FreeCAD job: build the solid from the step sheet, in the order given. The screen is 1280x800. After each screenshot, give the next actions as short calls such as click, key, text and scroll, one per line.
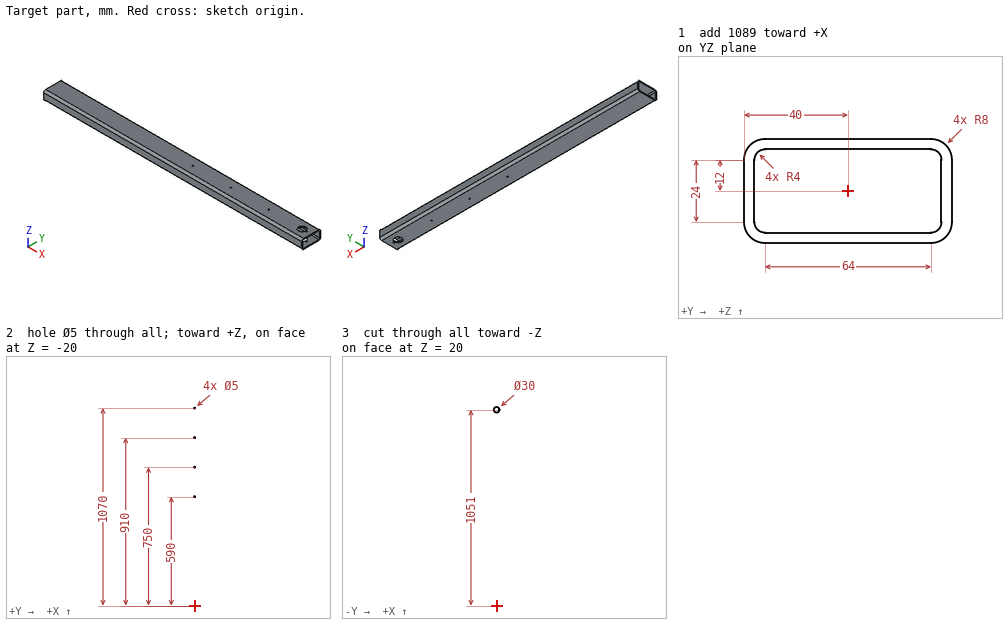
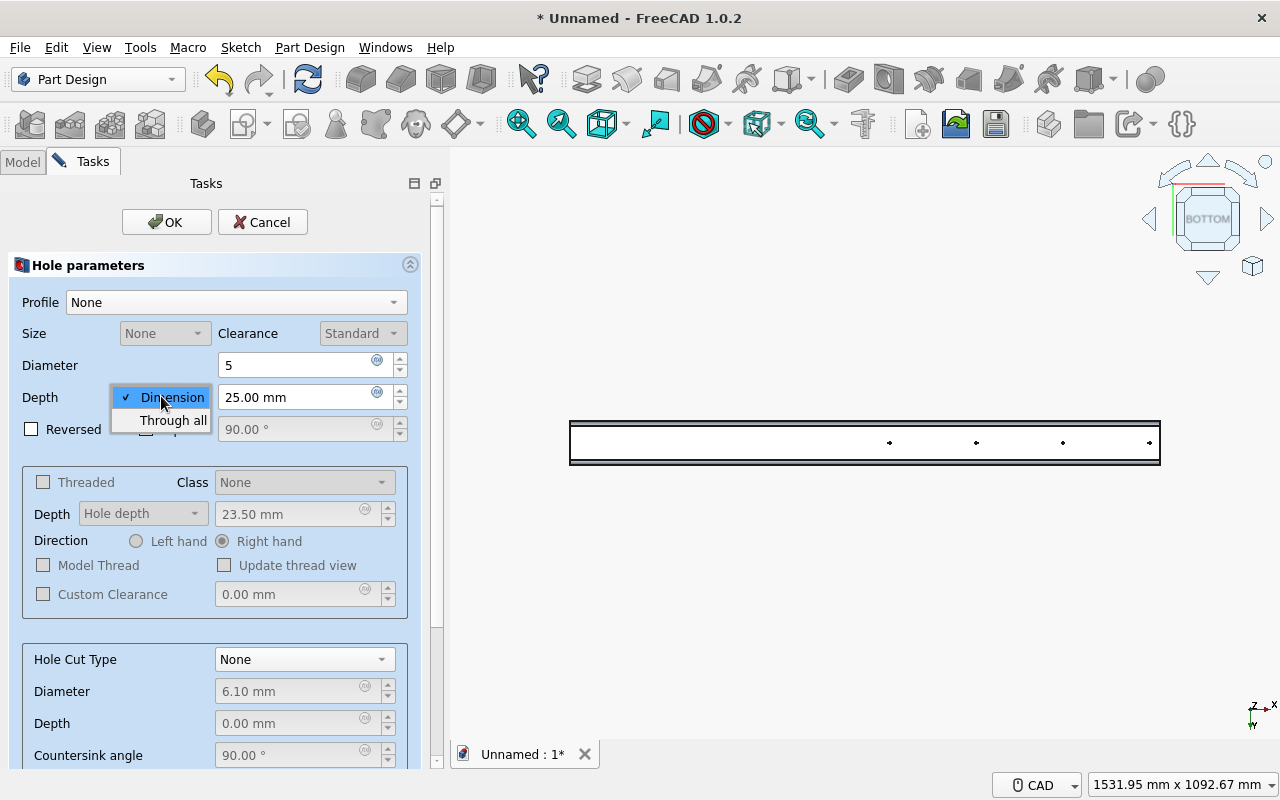
click(160, 420)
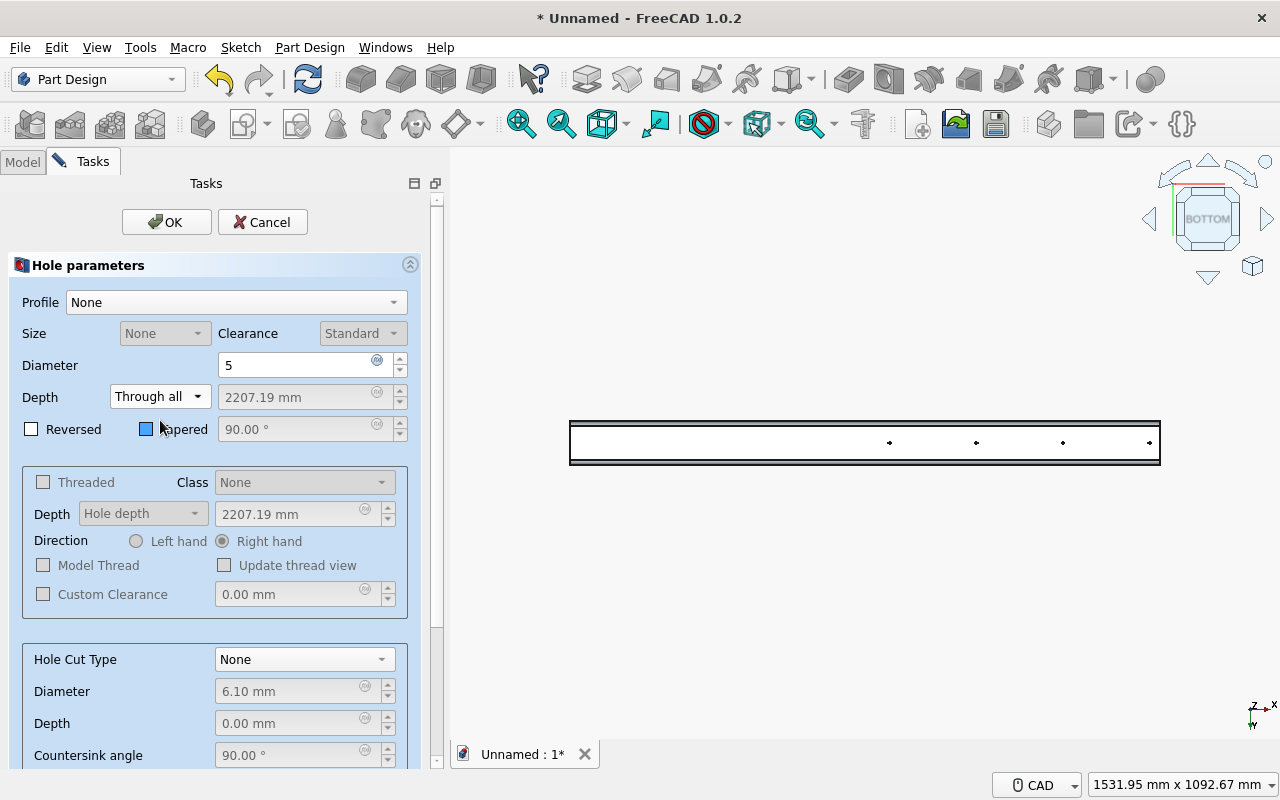
click(167, 222)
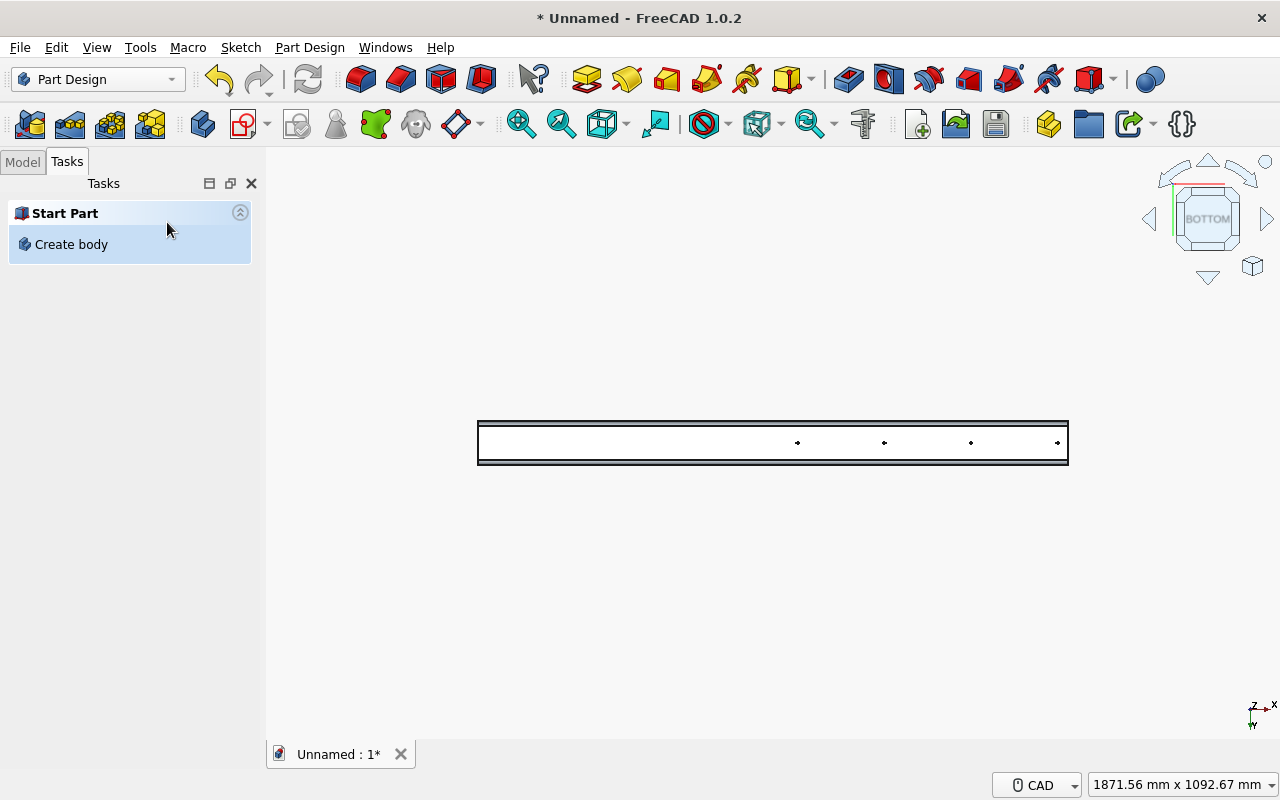
key(0)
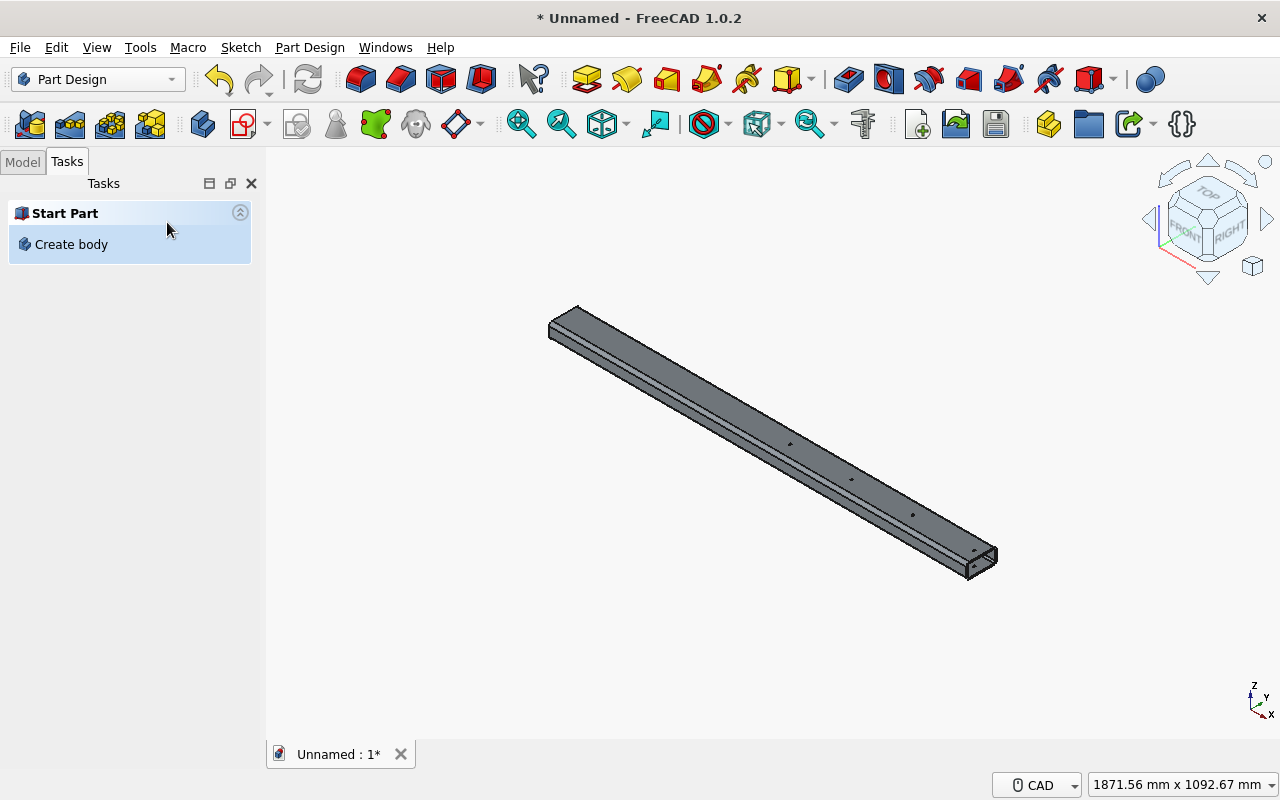
click(773, 433)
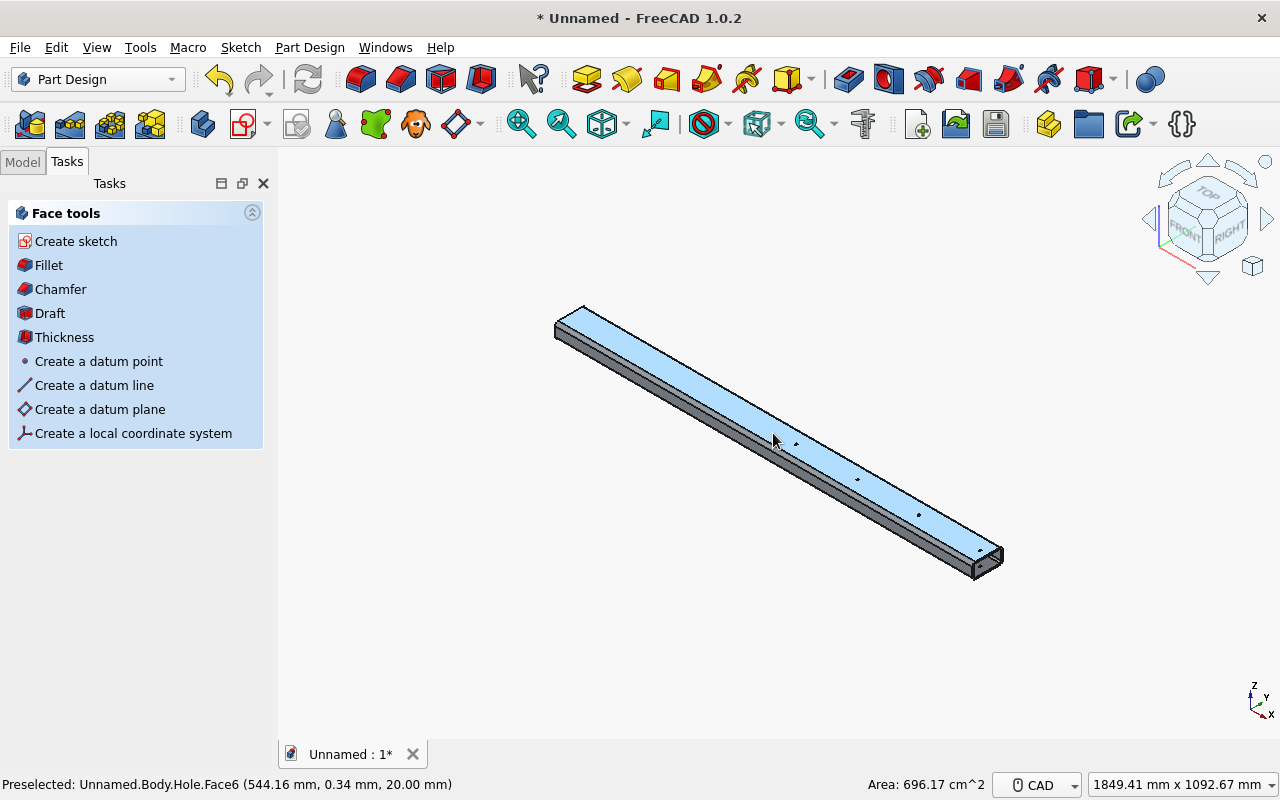
click(244, 124)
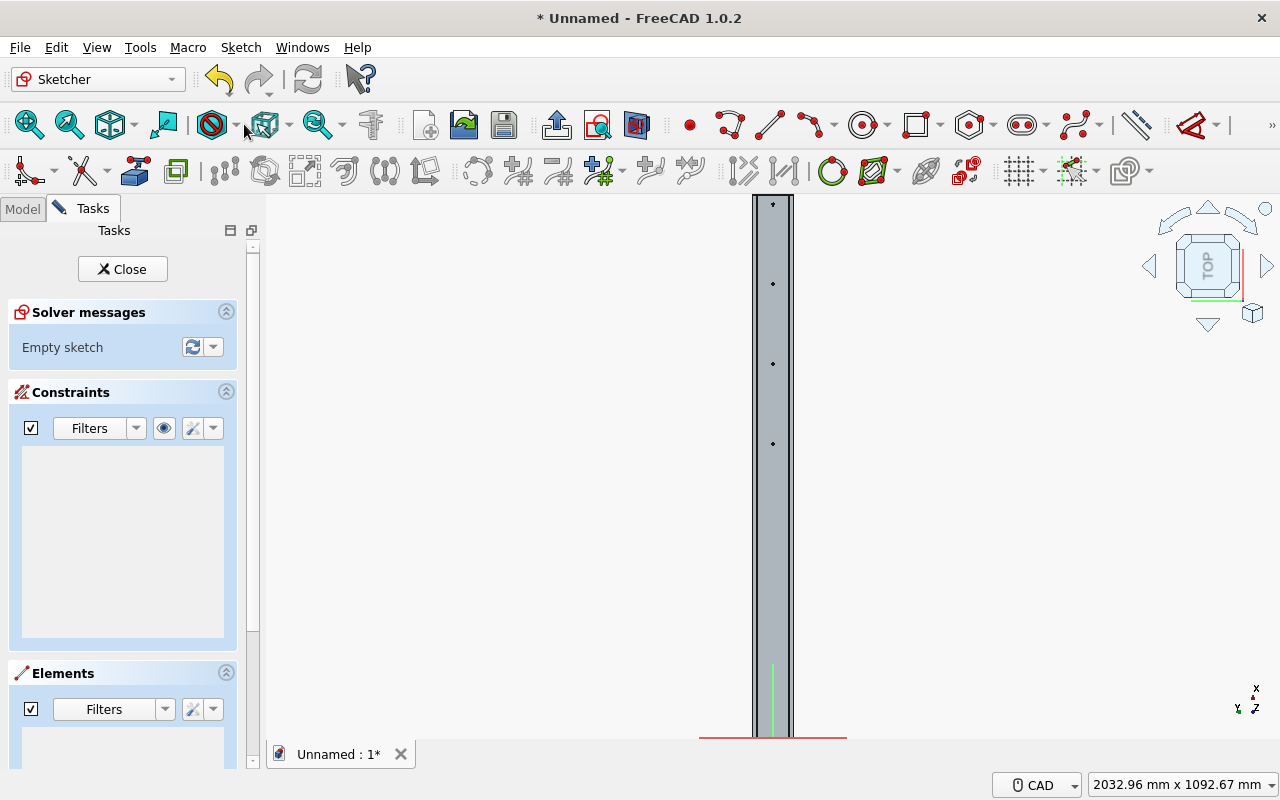
scroll(704, 466, down, 5)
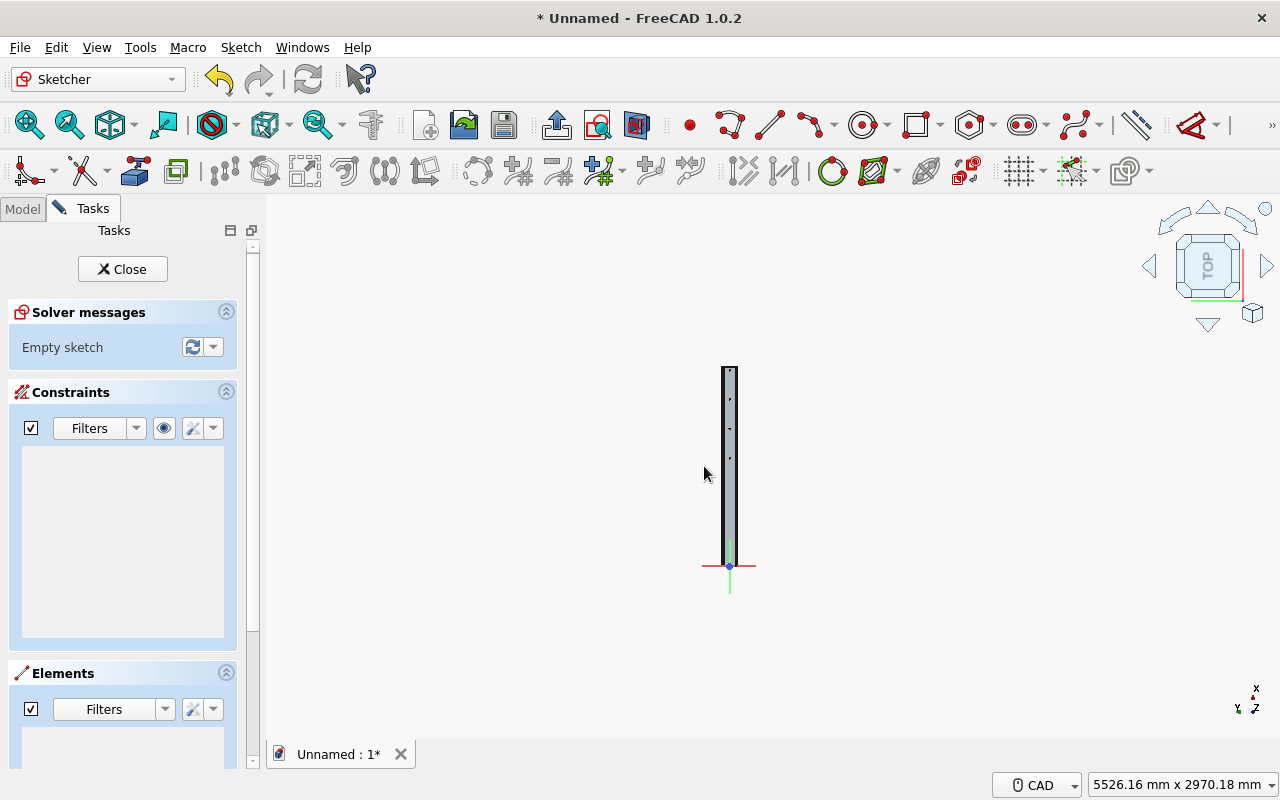
scroll(731, 369, up, 15)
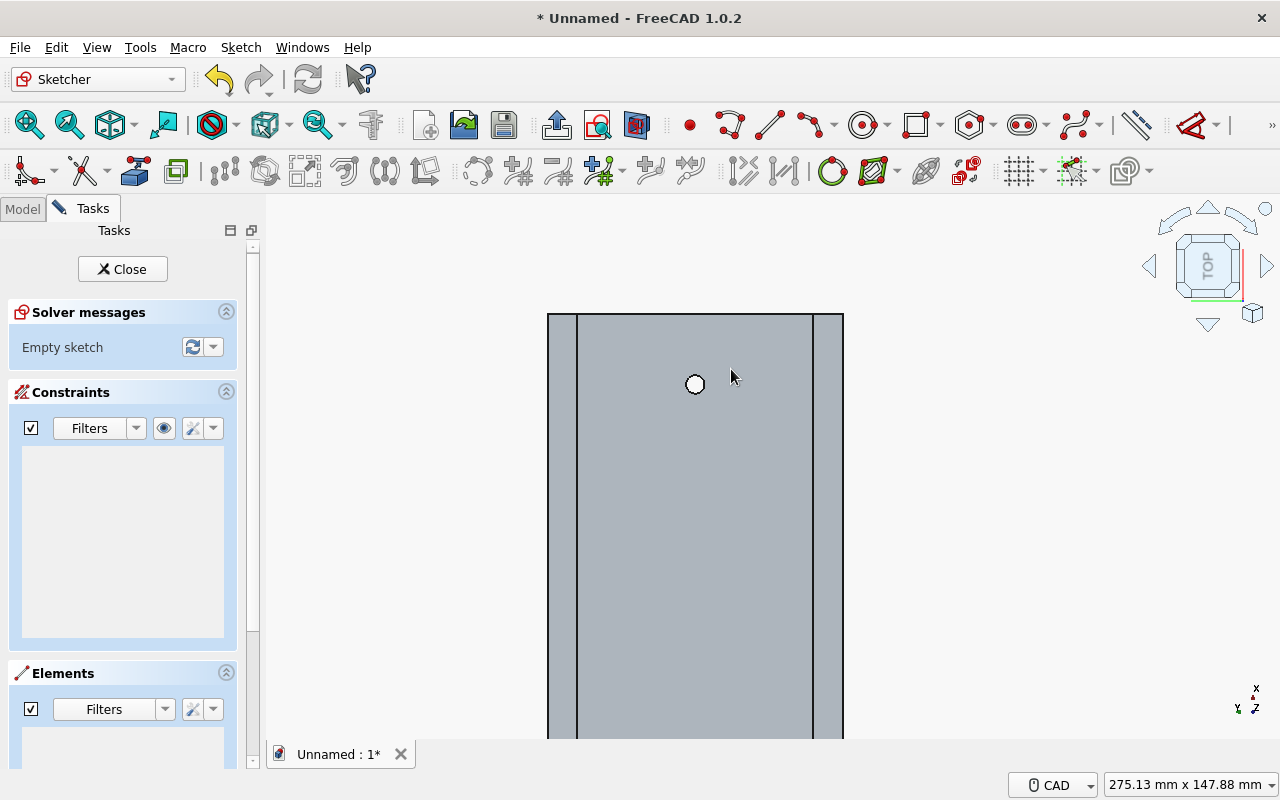
scroll(691, 449, up, 6)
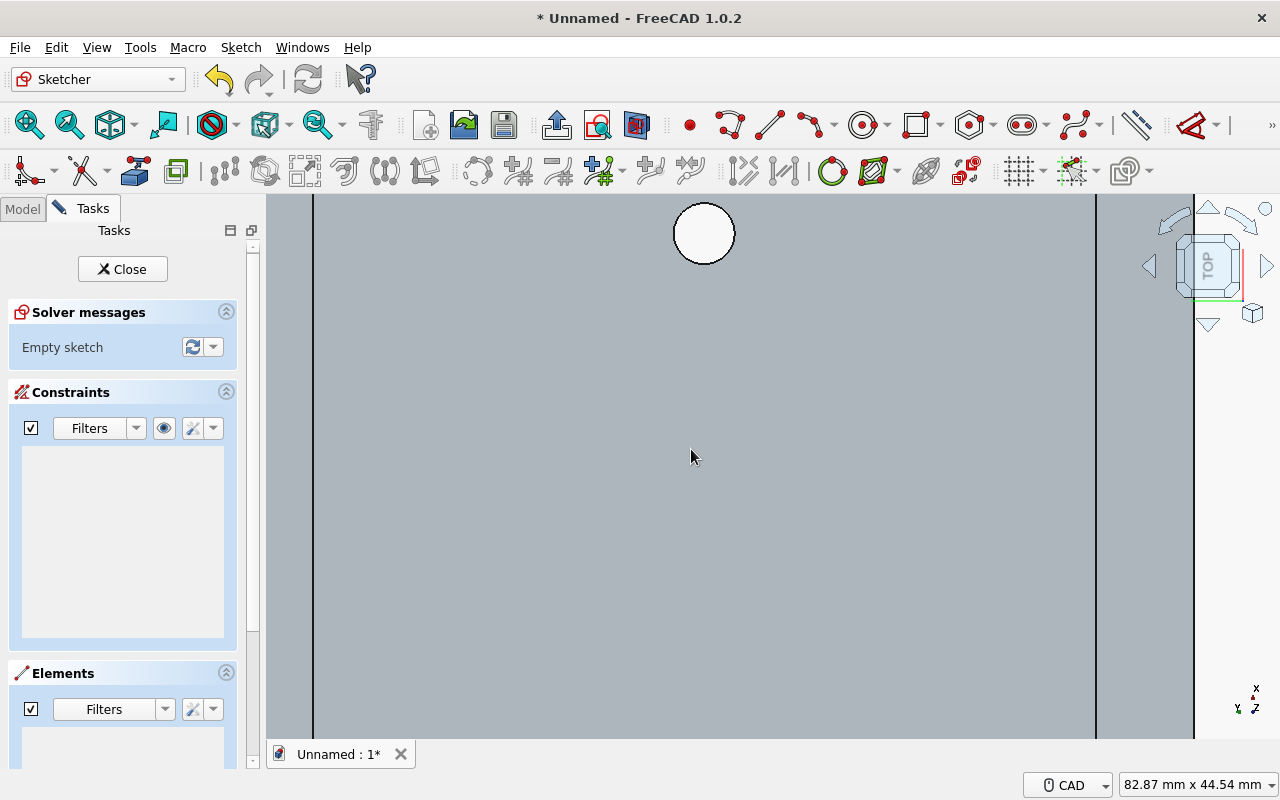
click(864, 126)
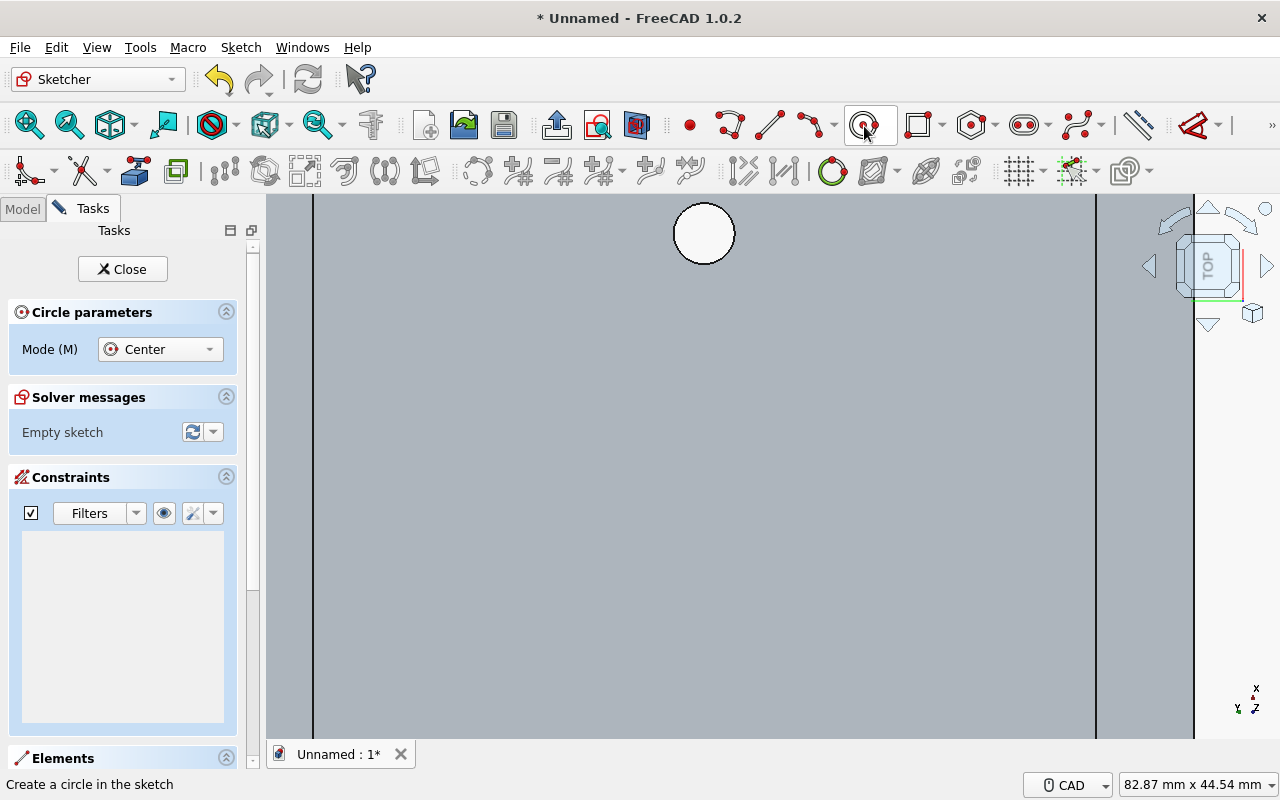
click(704, 466)
move(834, 336)